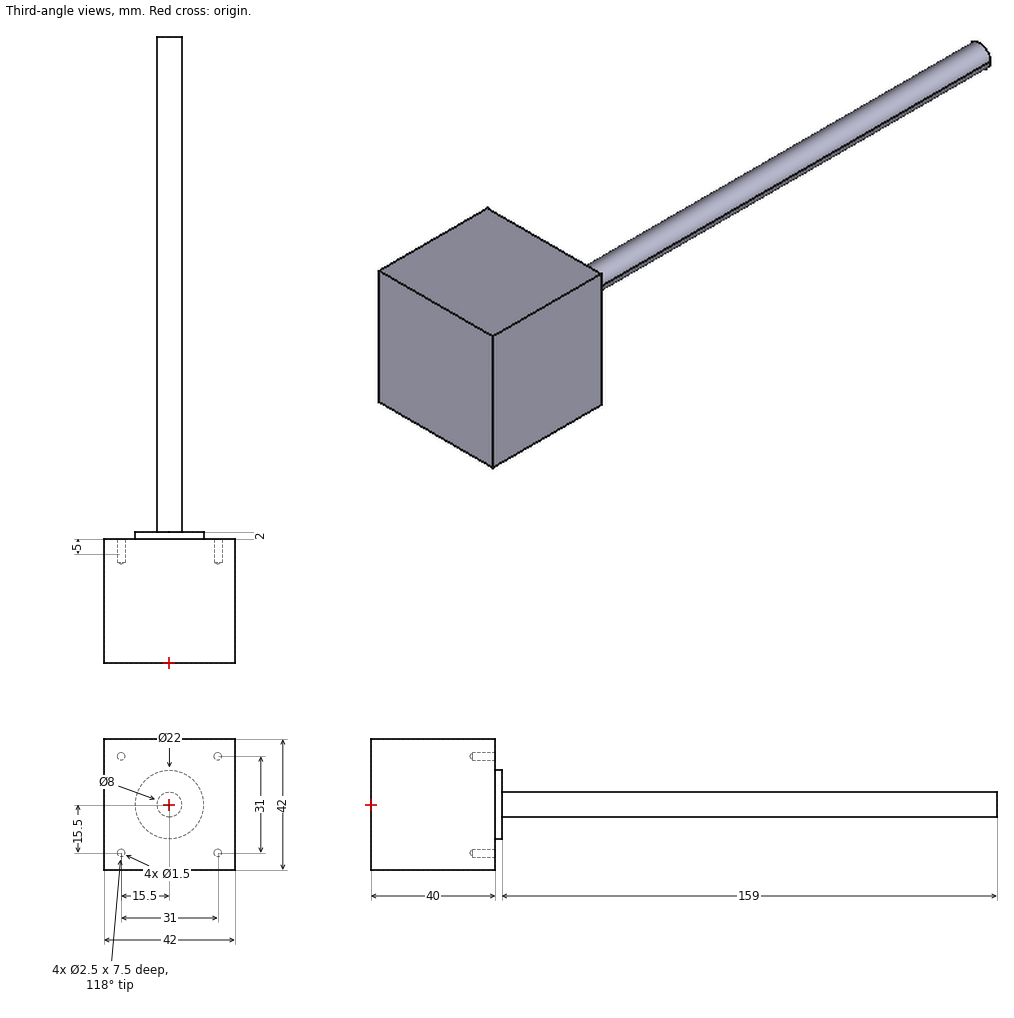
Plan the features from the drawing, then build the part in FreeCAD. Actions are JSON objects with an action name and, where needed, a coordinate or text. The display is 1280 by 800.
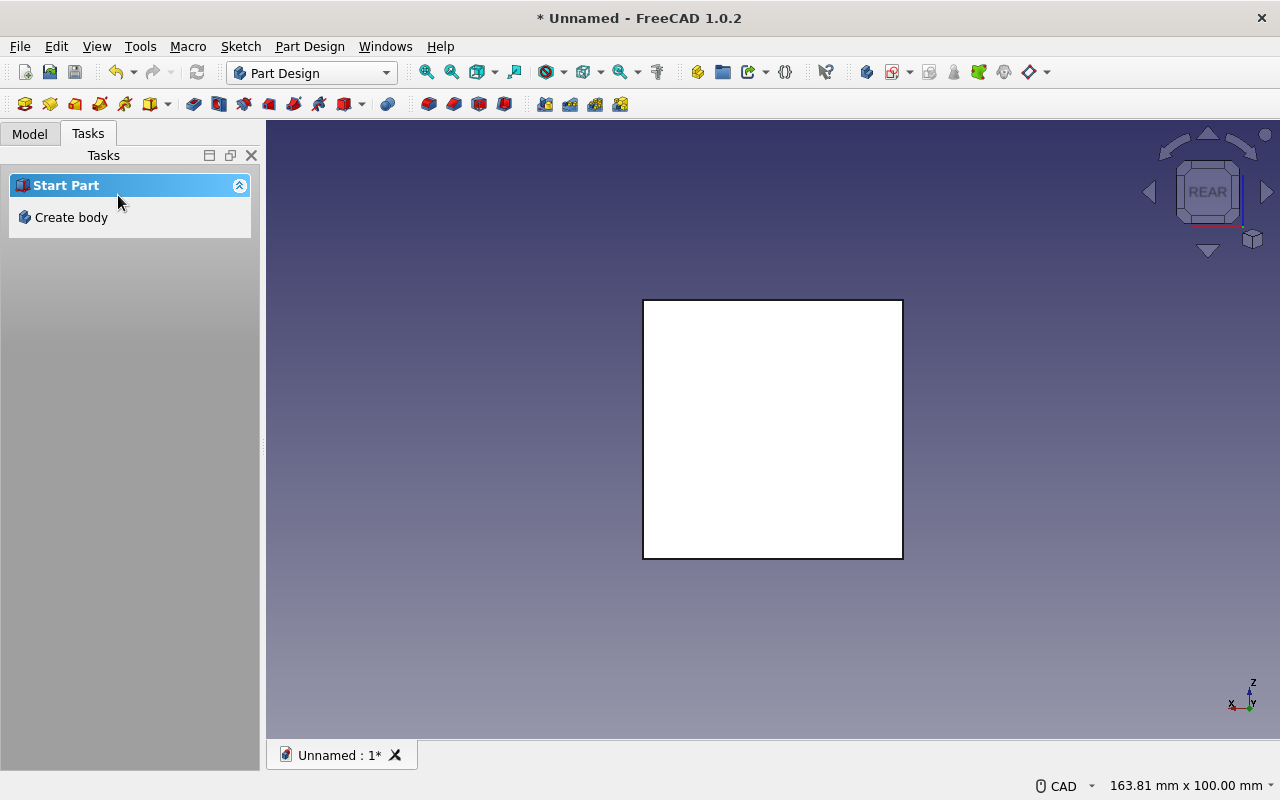
{"action": "key", "text": "v f"}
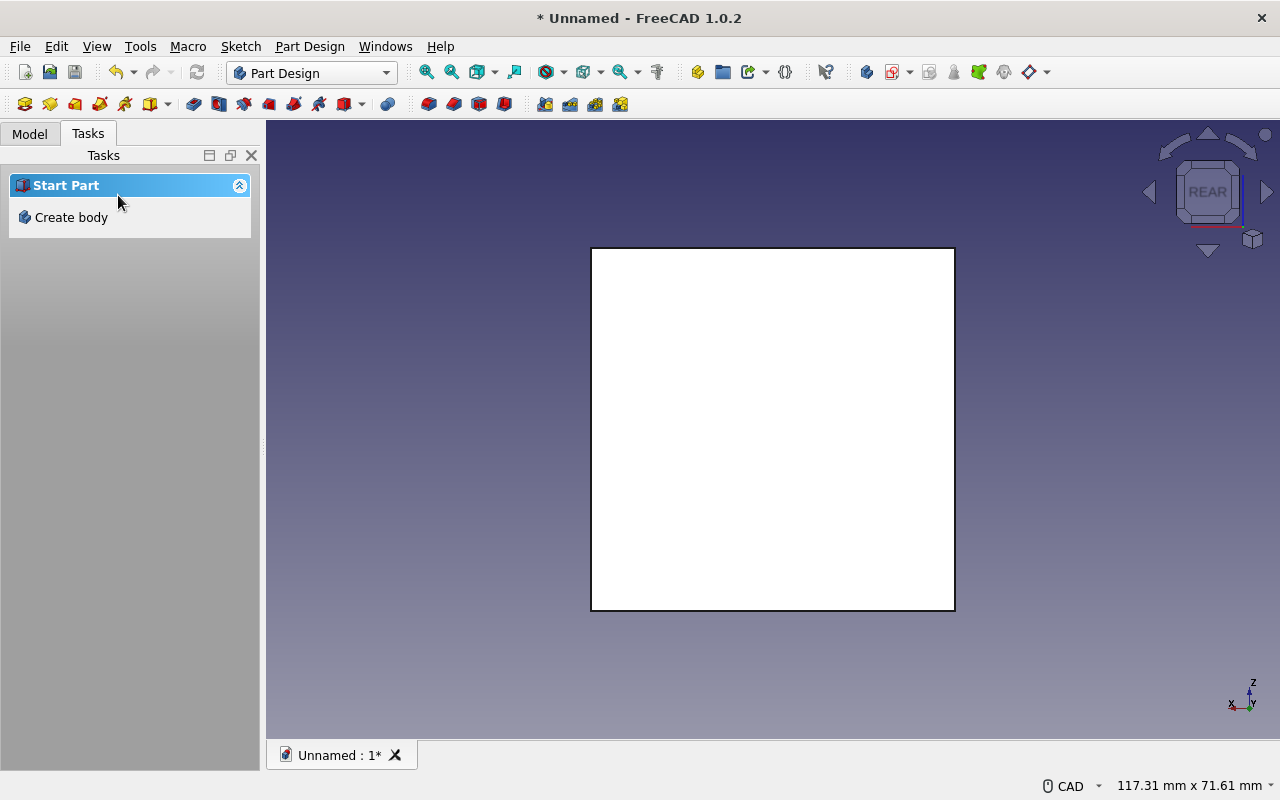
{"action": "left_click", "coordinate": [773, 429]}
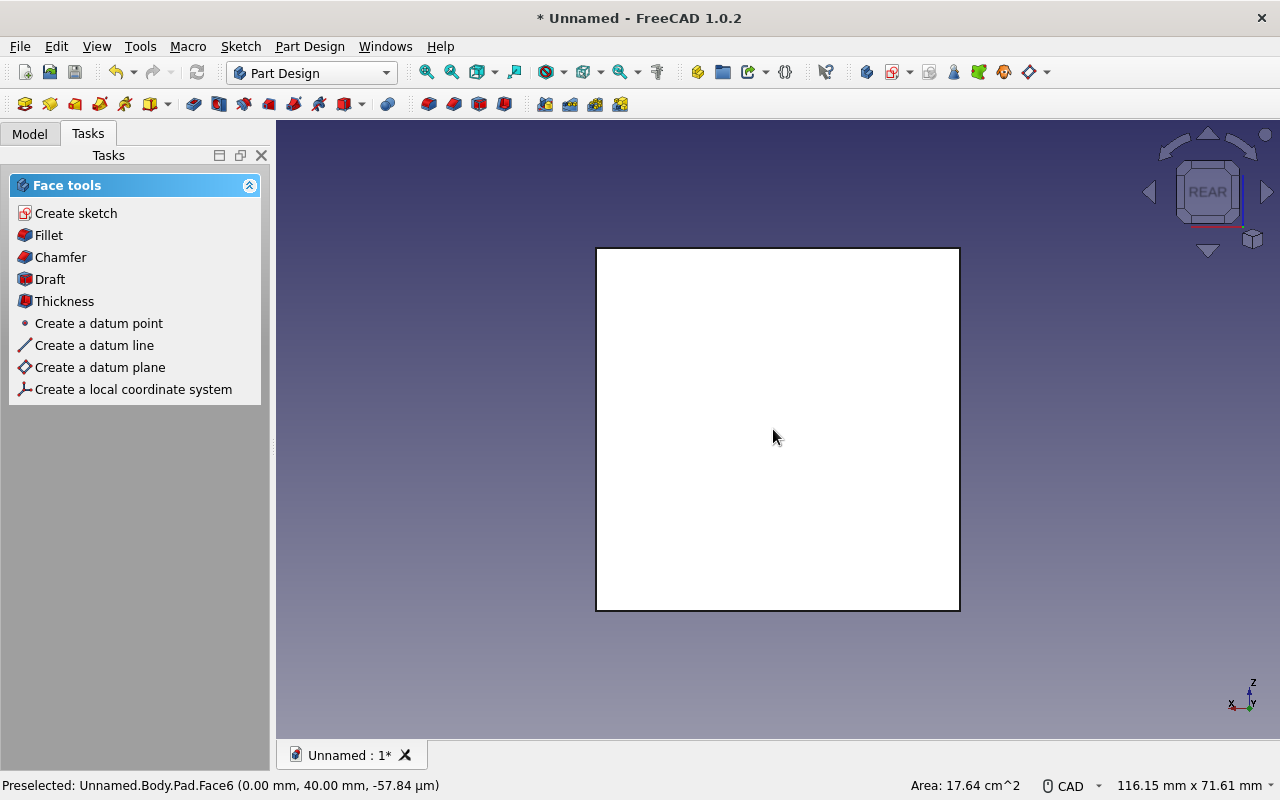
{"action": "left_click", "coordinate": [892, 72]}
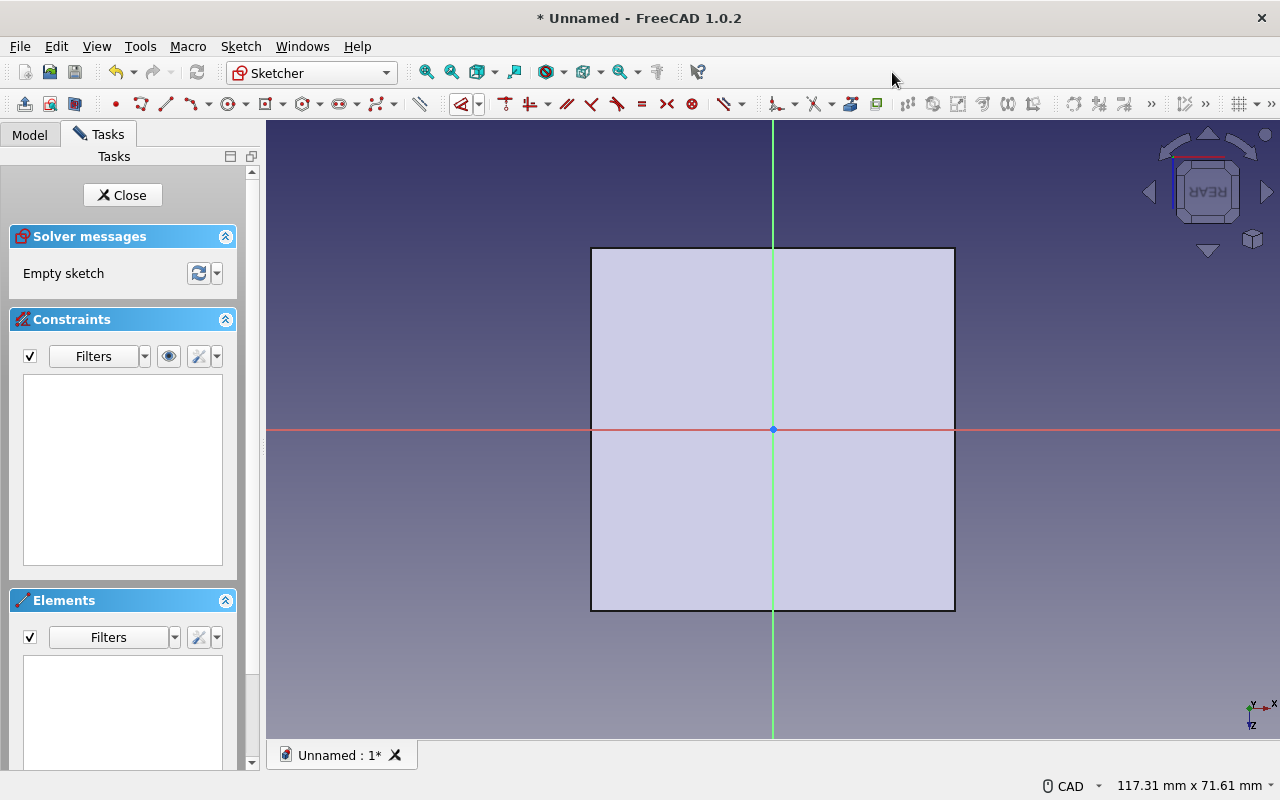
{"action": "scroll", "coordinate": [829, 429], "scroll_direction": "up", "scroll_amount": 4}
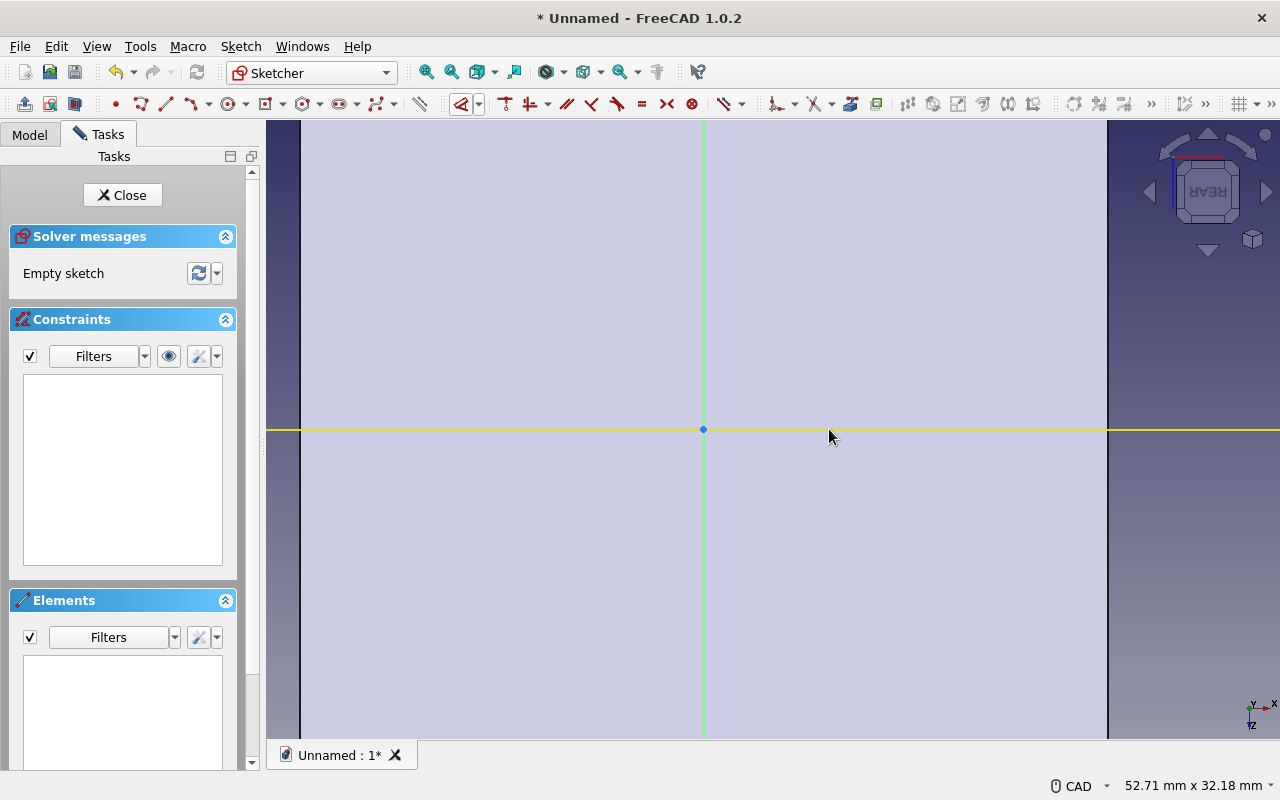
{"action": "left_click", "coordinate": [228, 104]}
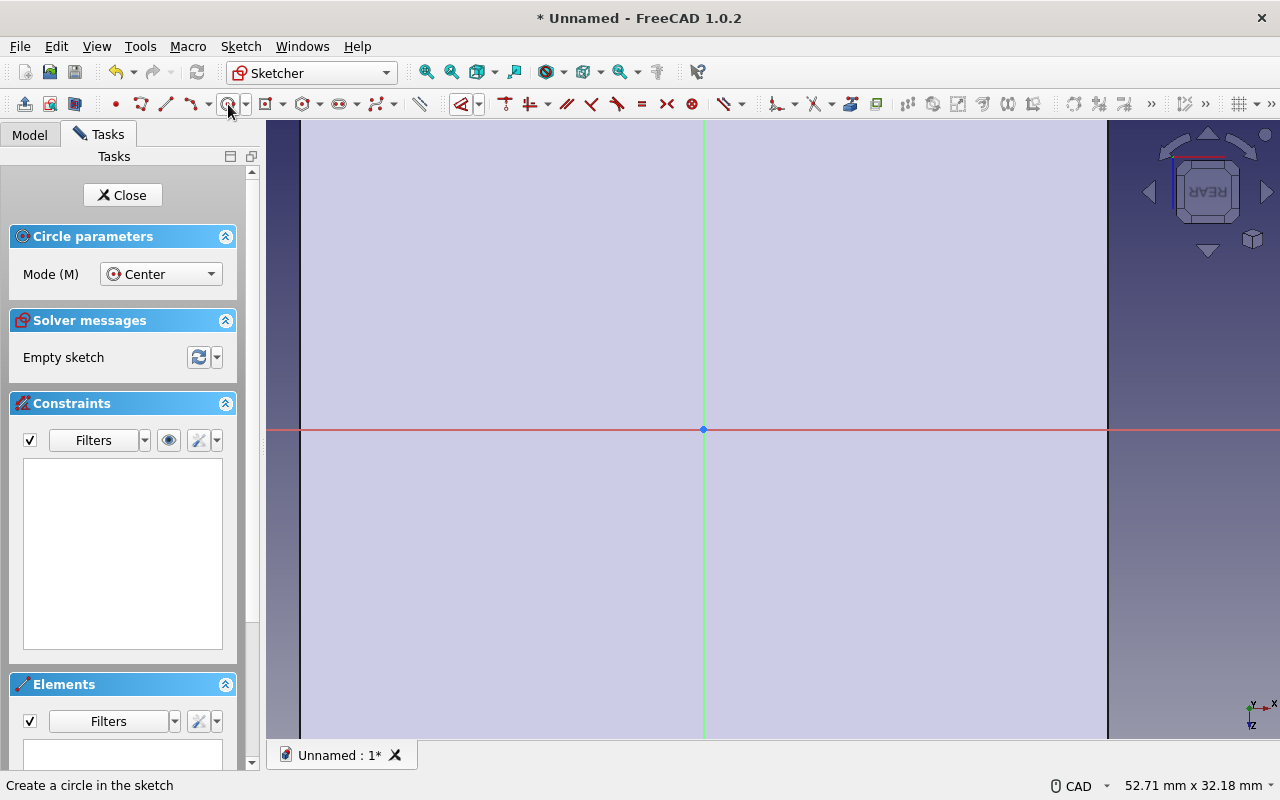
{"action": "left_click", "coordinate": [704, 429]}
{"action": "left_click", "coordinate": [853, 280]}
{"action": "key", "text": "Escape"}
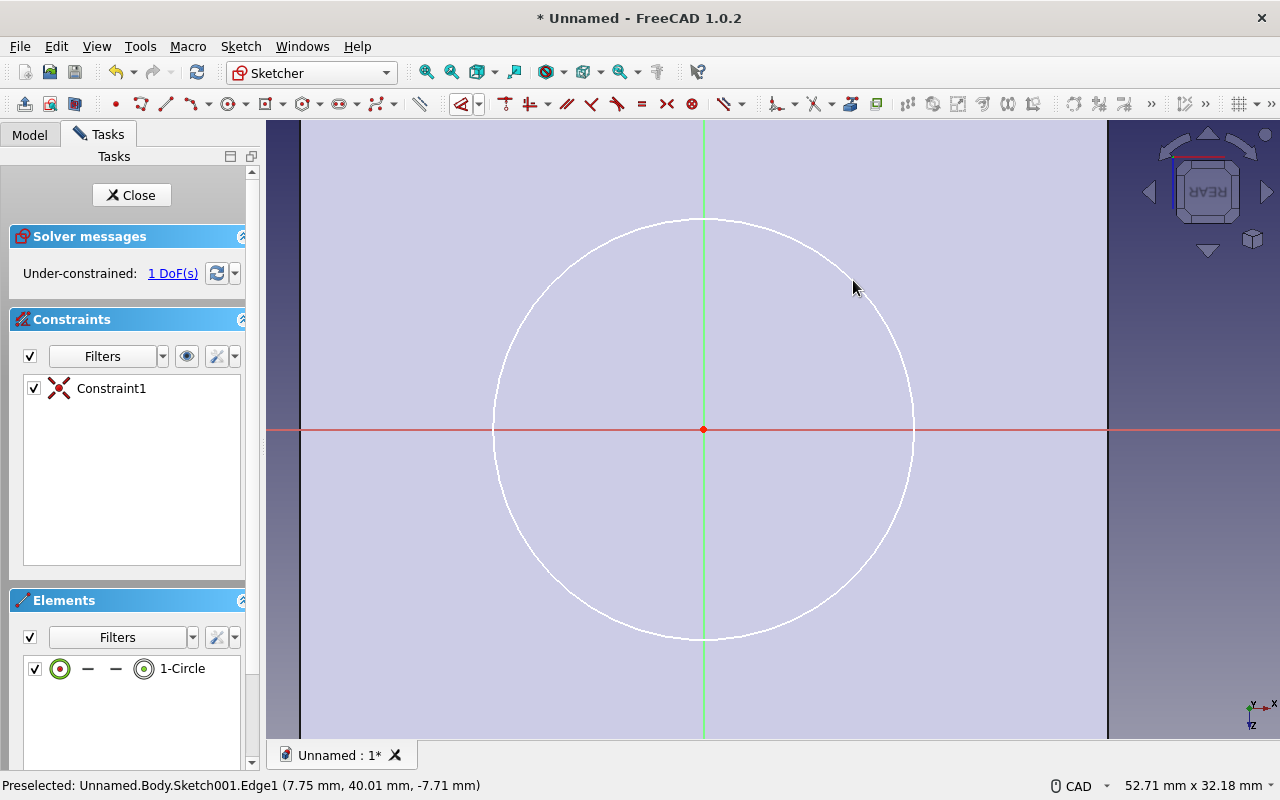
{"action": "left_click", "coordinate": [852, 280]}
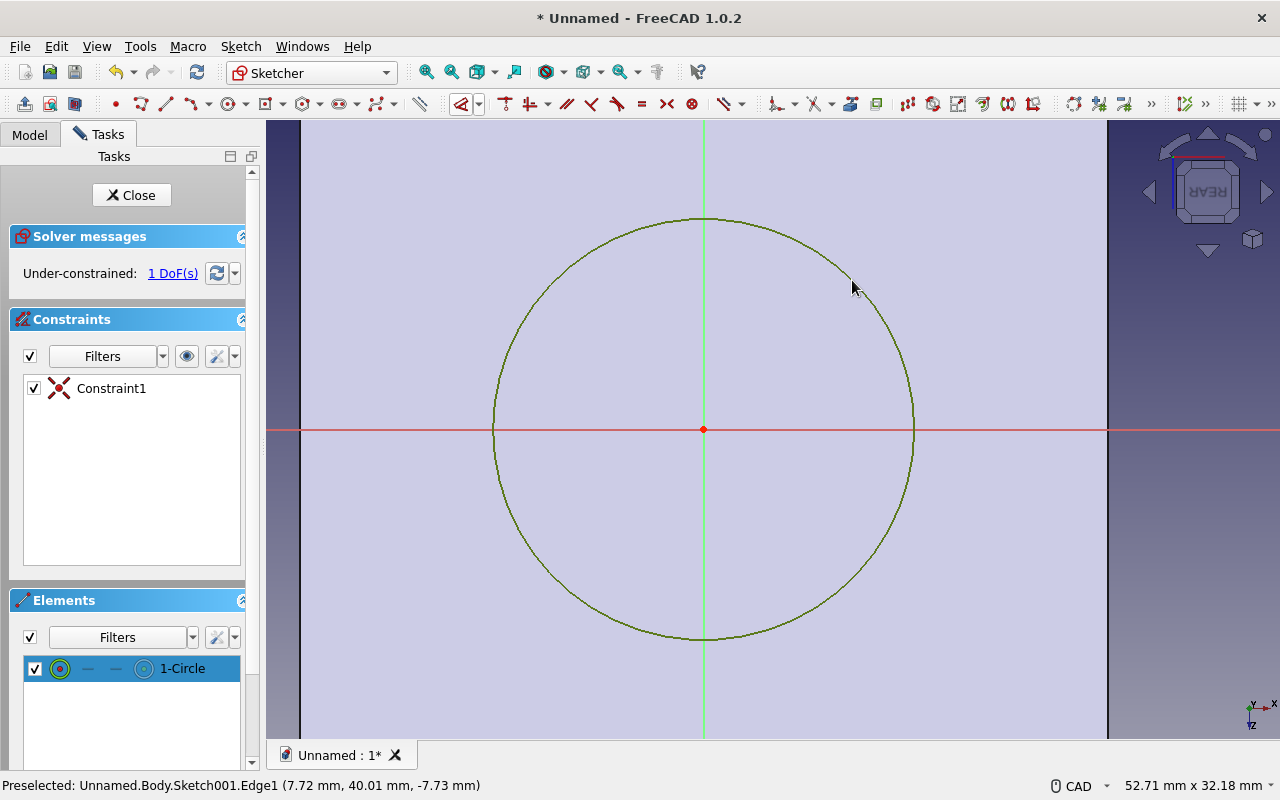
{"action": "left_click", "coordinate": [478, 104]}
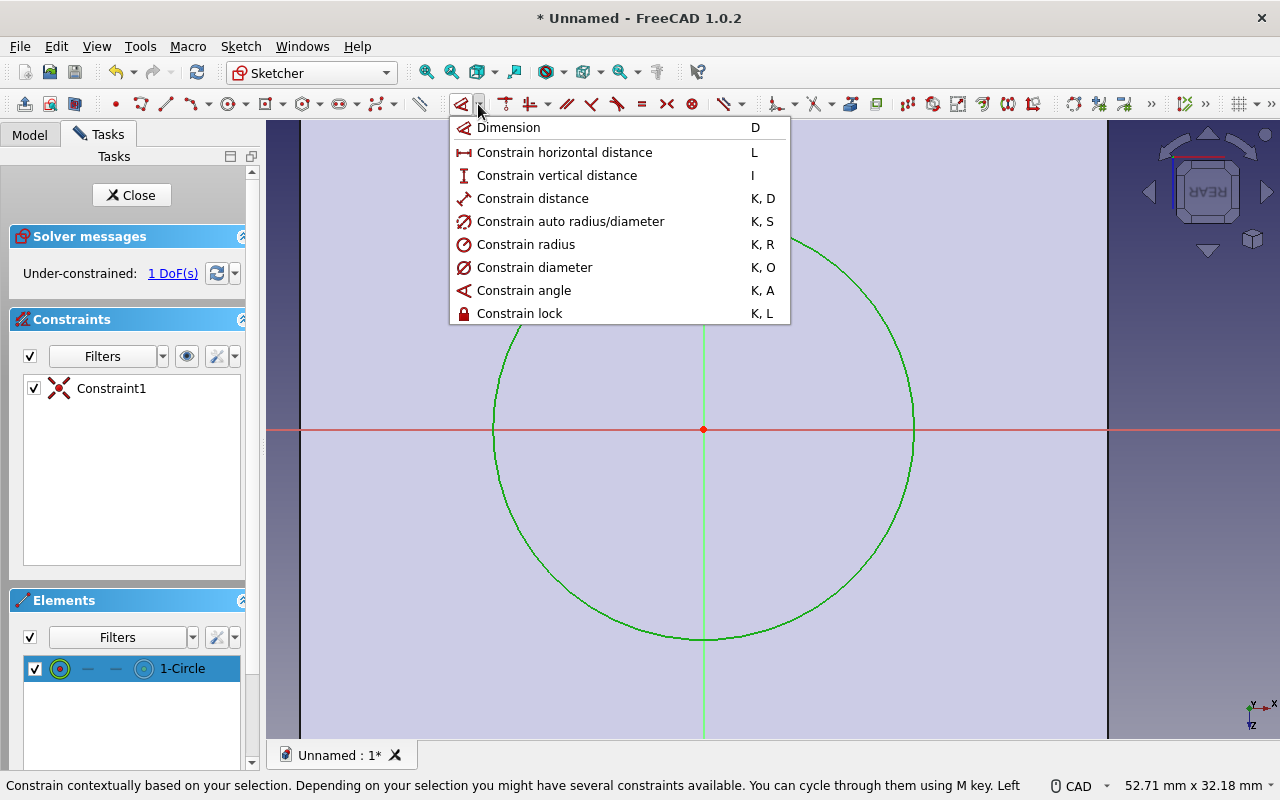
{"action": "left_click", "coordinate": [620, 268]}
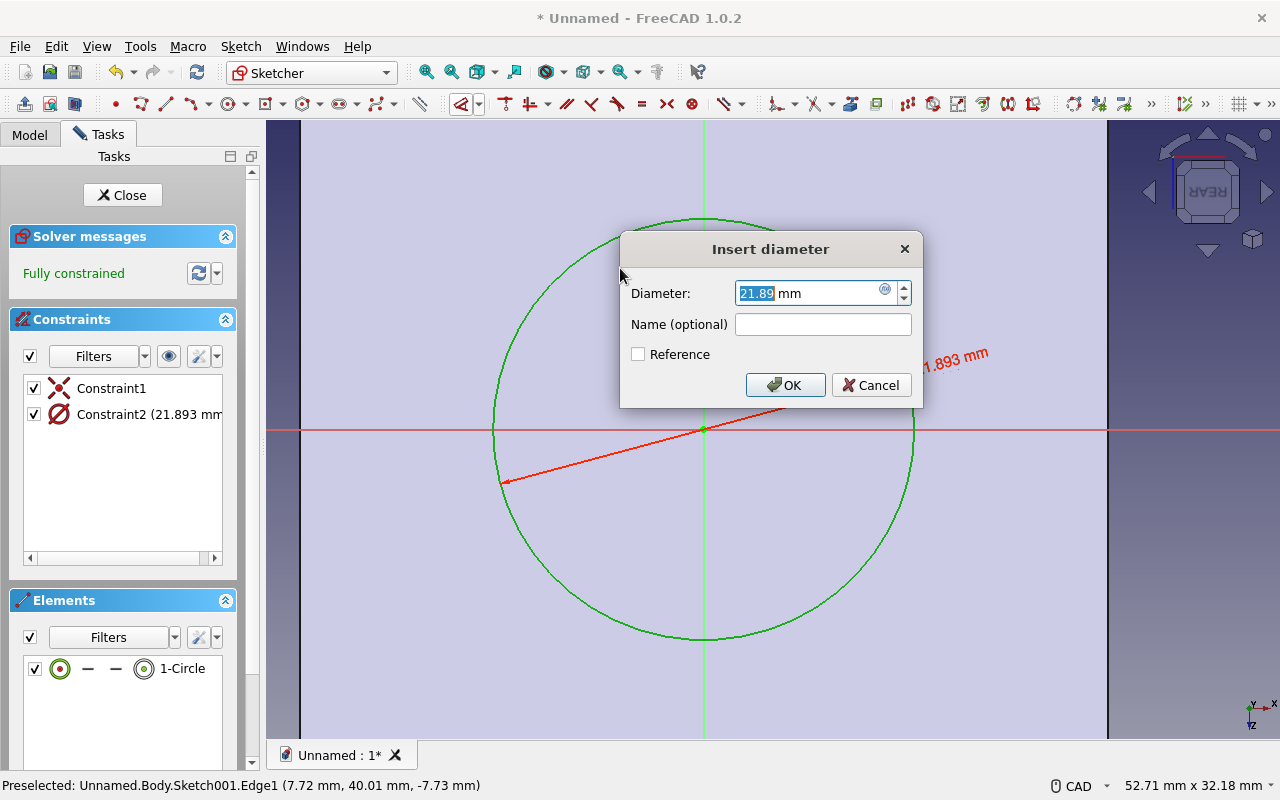
{"action": "type", "text": "22"}
{"action": "key", "text": "Return"}